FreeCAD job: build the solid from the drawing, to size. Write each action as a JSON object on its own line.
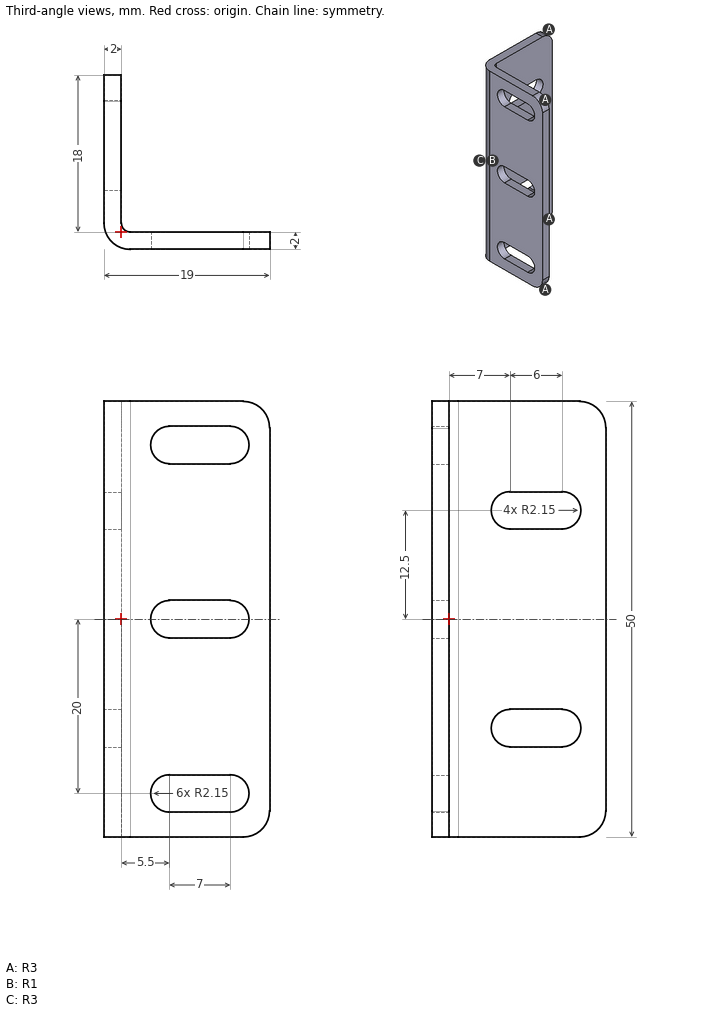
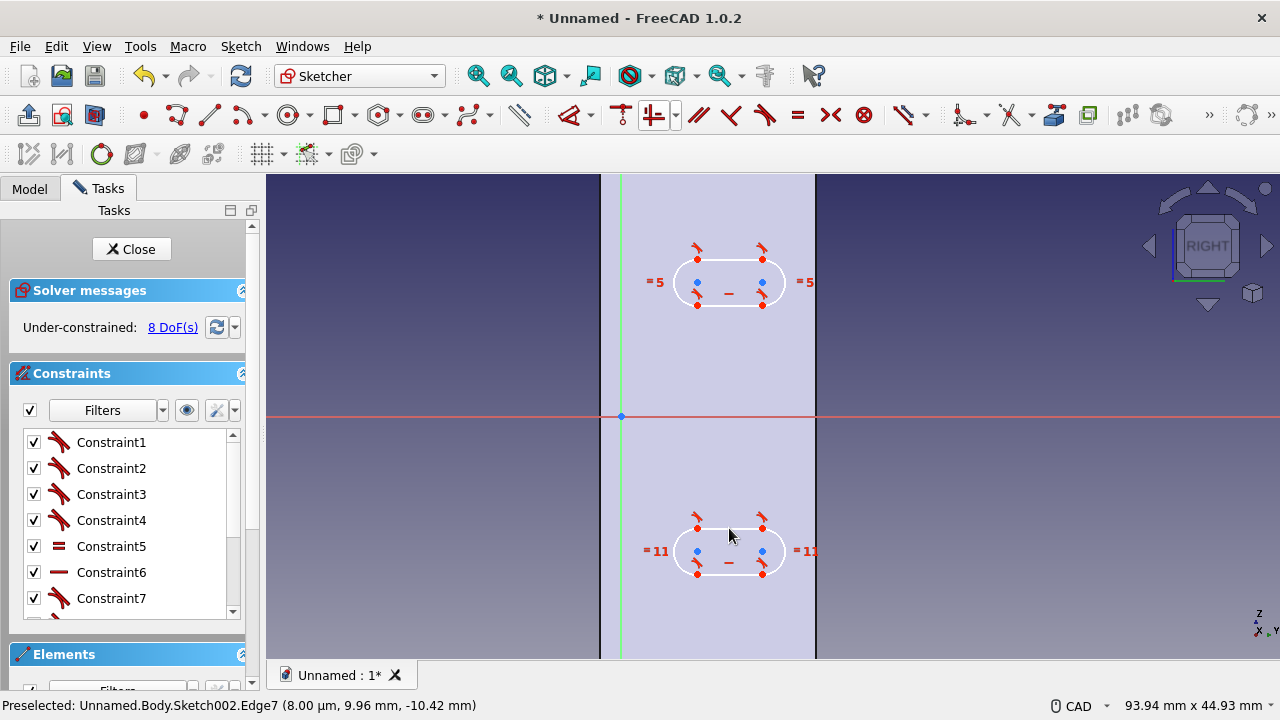
{"action": "left_click", "coordinate": [678, 269]}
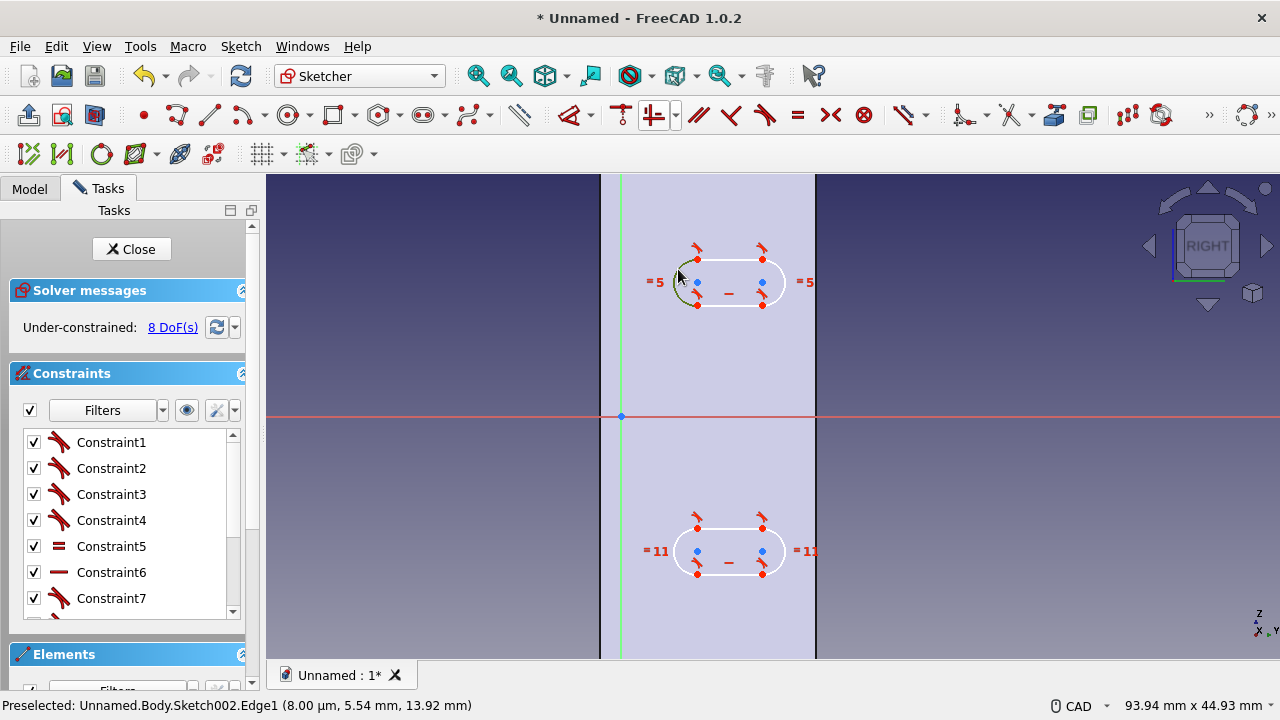
{"action": "left_click", "coordinate": [678, 538]}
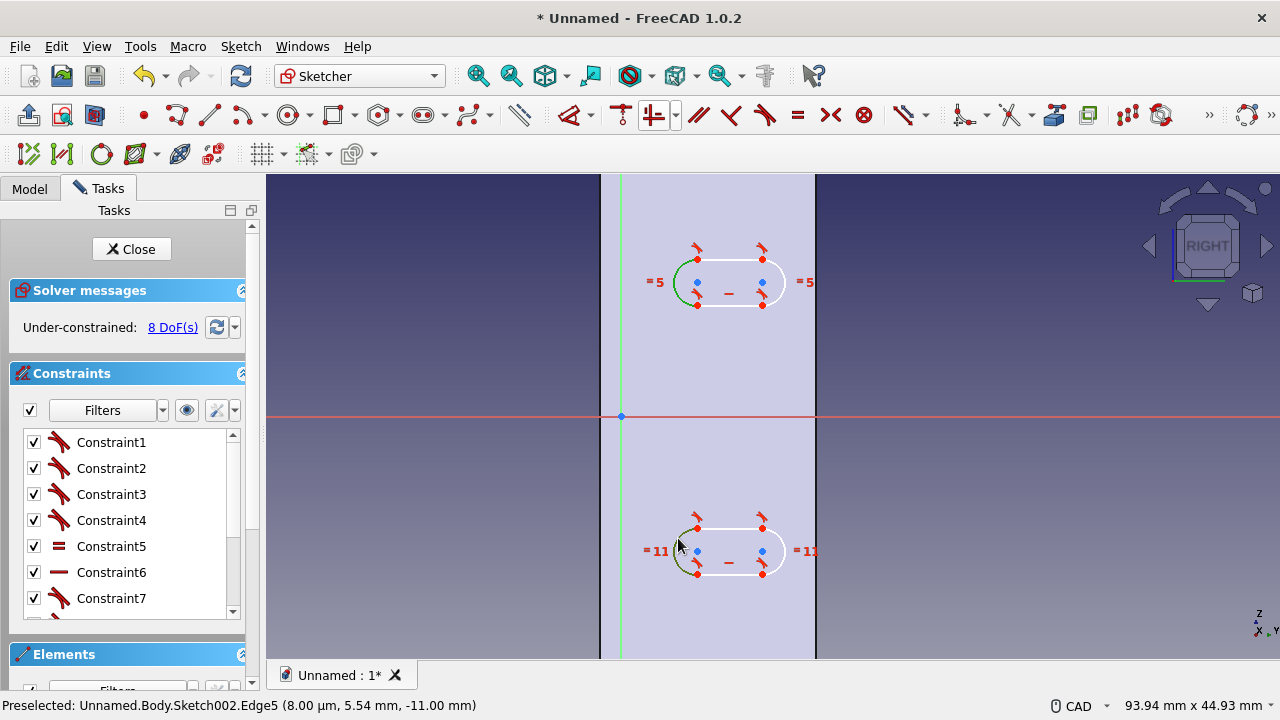
{"action": "left_click", "coordinate": [798, 116]}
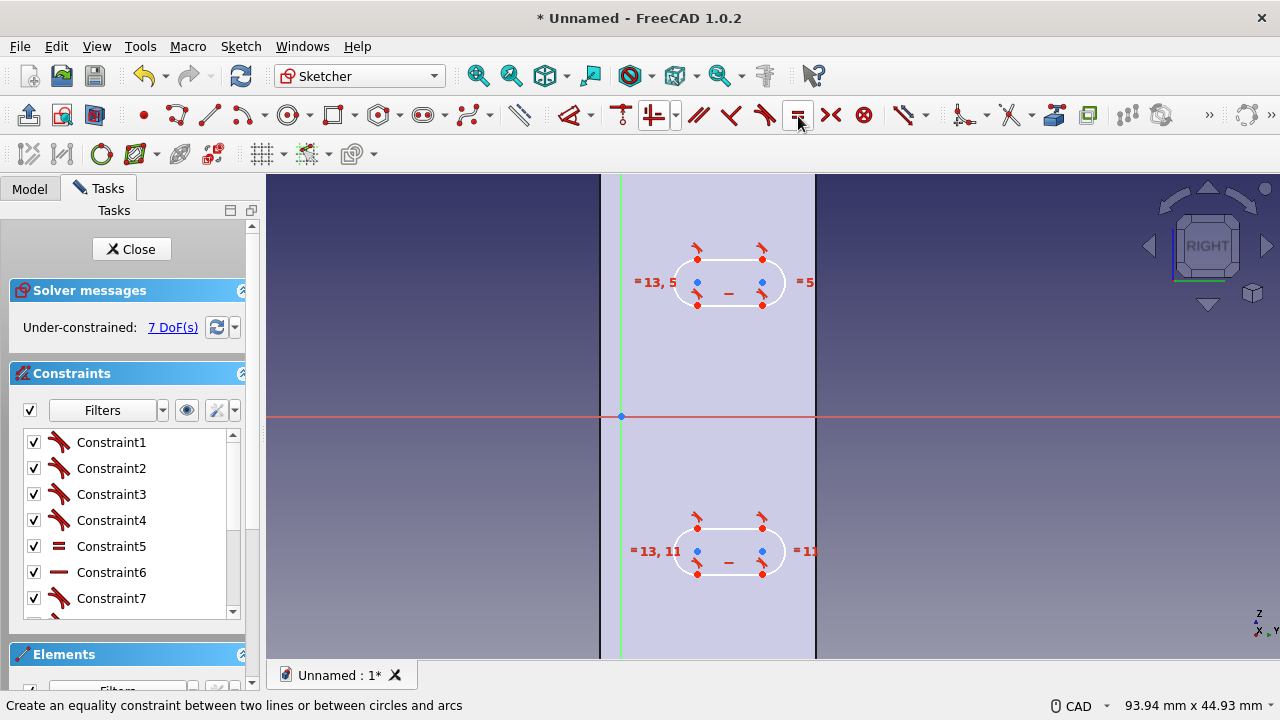
{"action": "left_click", "coordinate": [697, 283]}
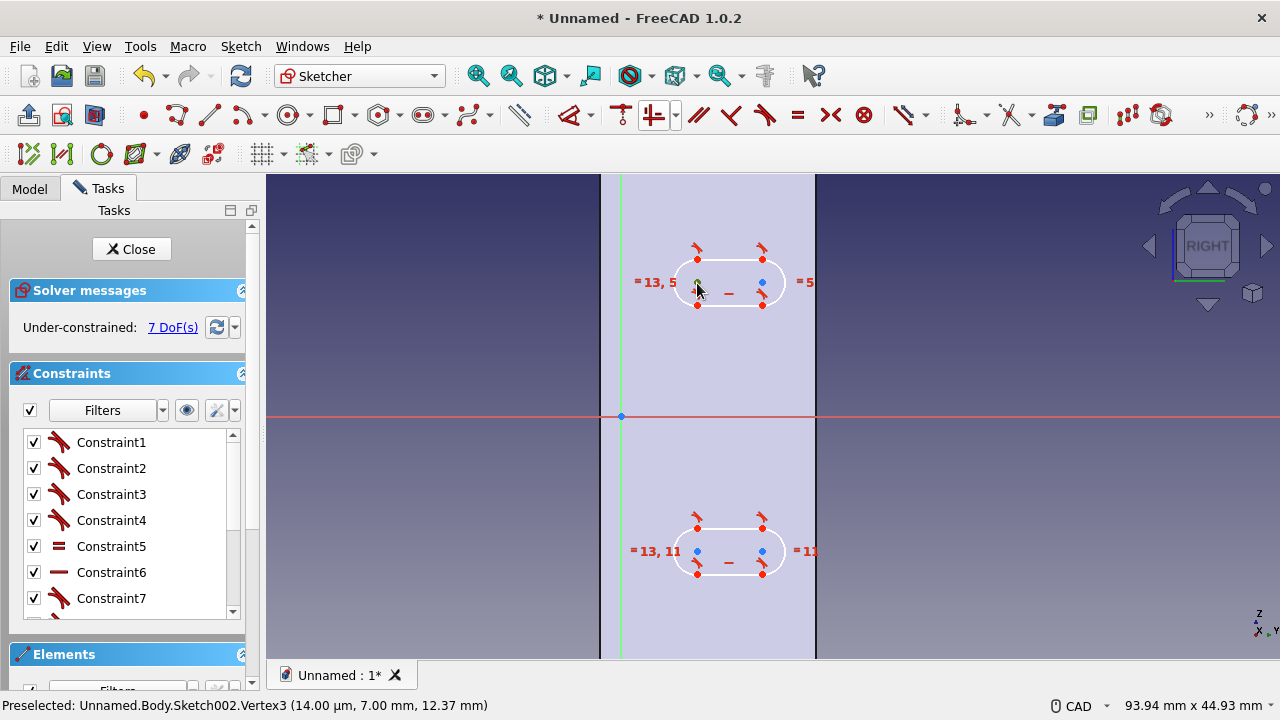
{"action": "left_click", "coordinate": [697, 552]}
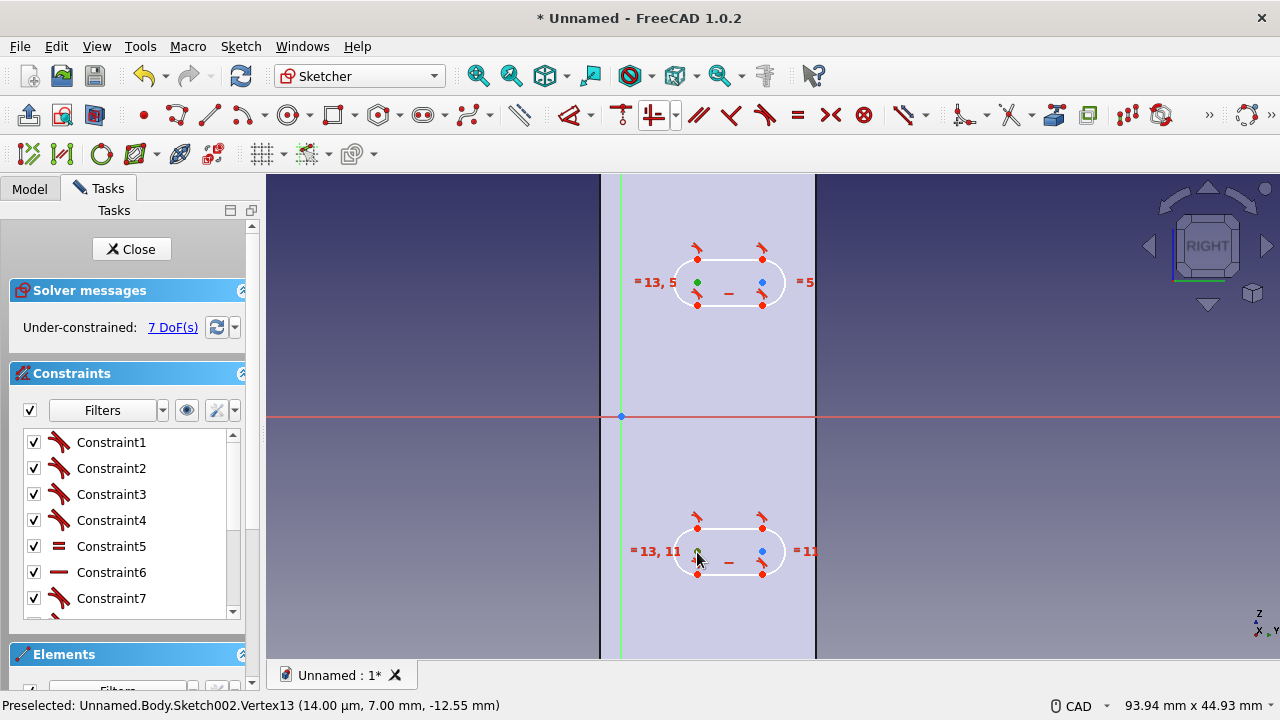
{"action": "left_click", "coordinate": [353, 416]}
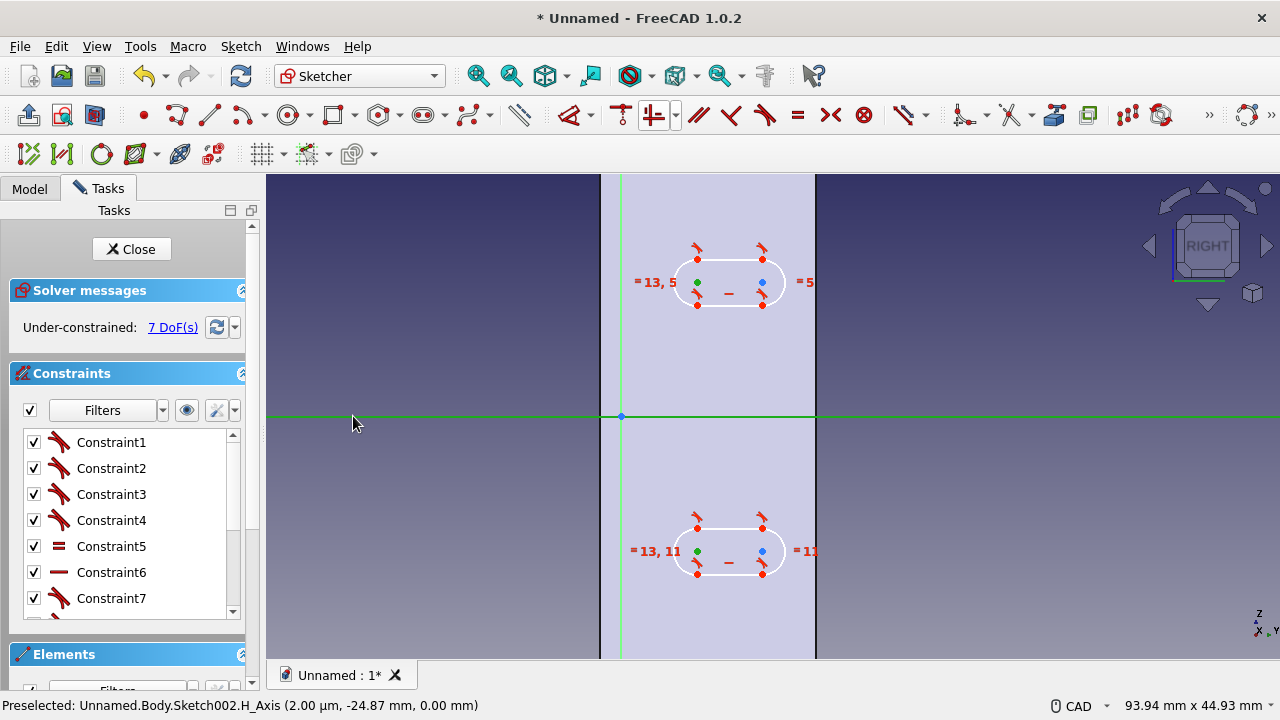
{"action": "left_click", "coordinate": [831, 116]}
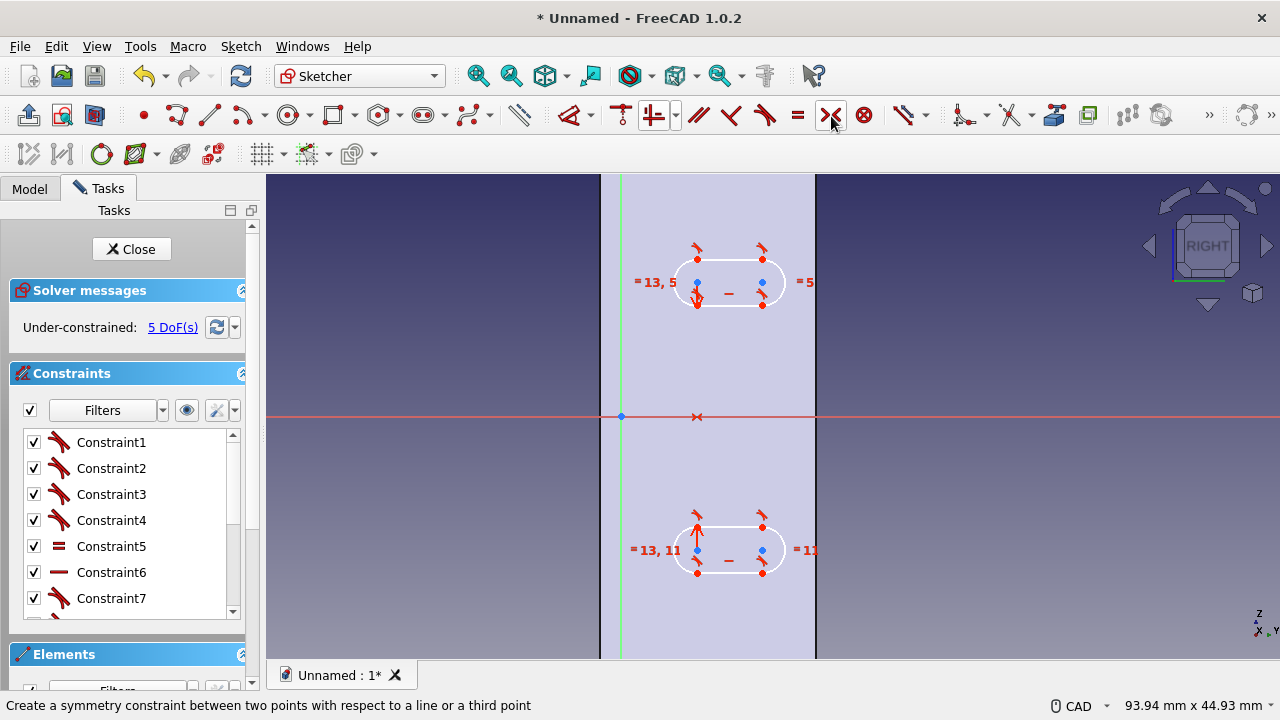
{"action": "left_click", "coordinate": [568, 116]}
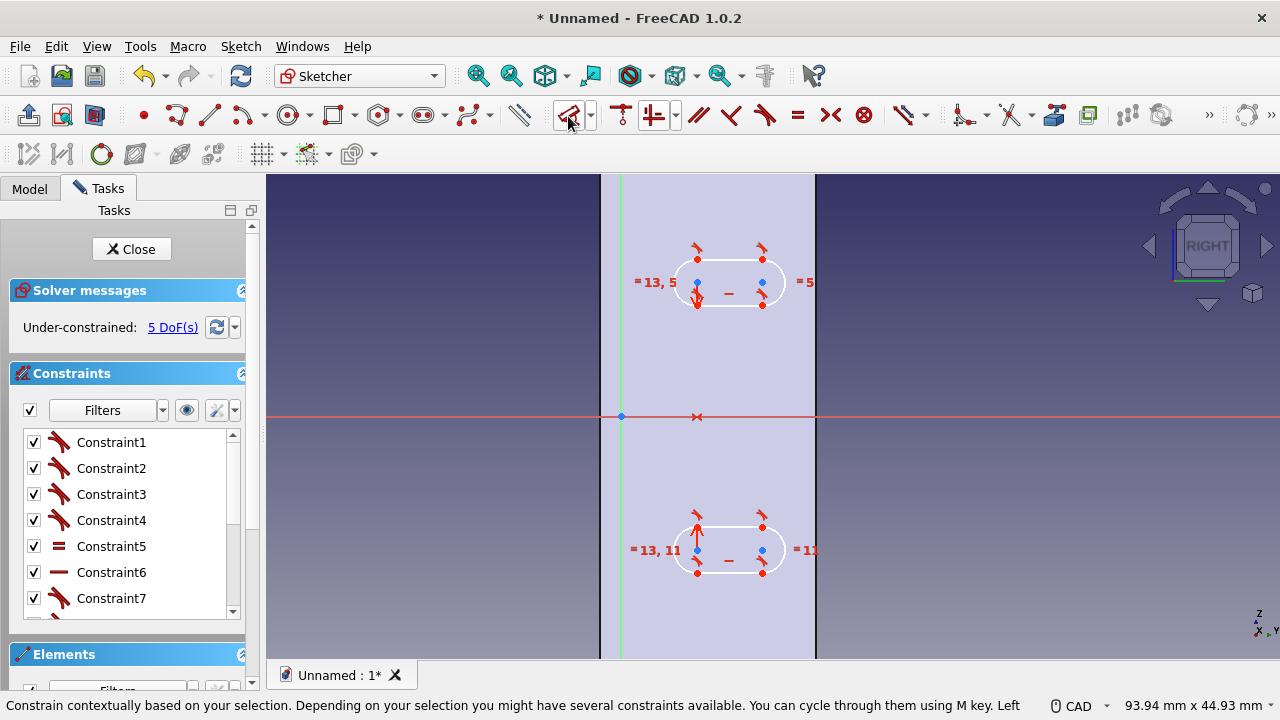
{"action": "scroll", "coordinate": [678, 269], "scroll_direction": "up", "scroll_amount": 3}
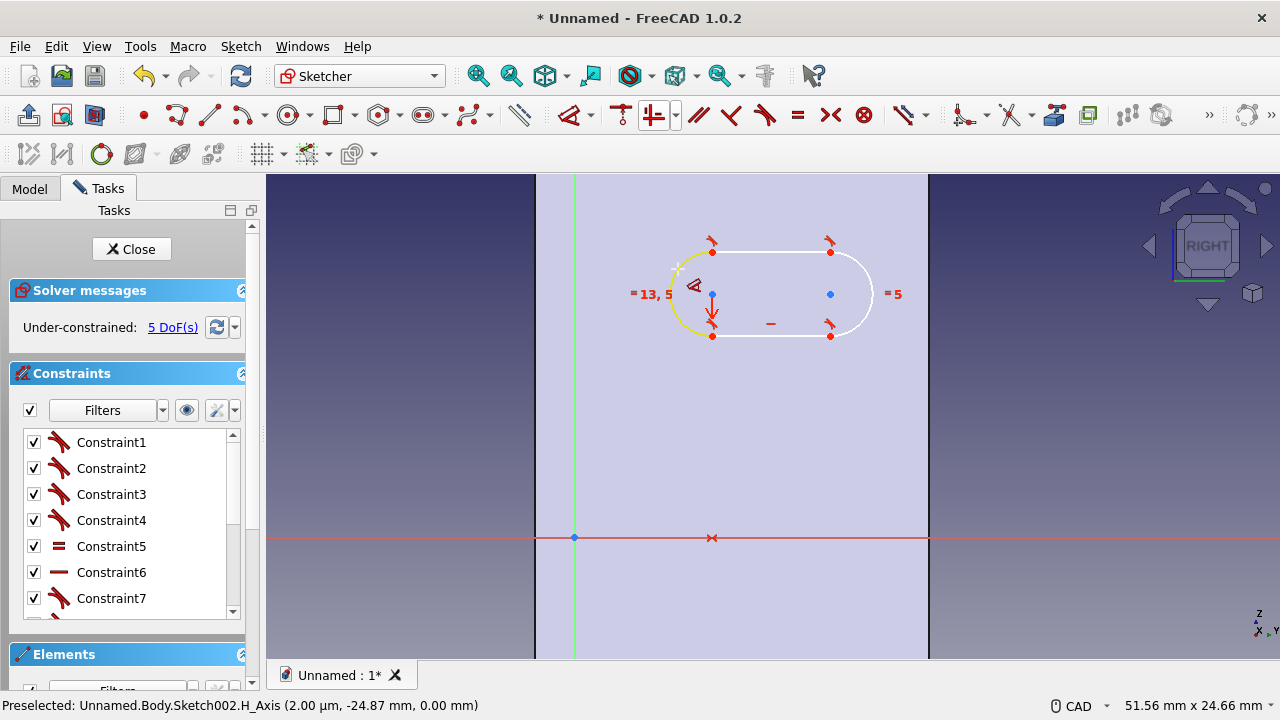
{"action": "left_click", "coordinate": [678, 270]}
{"action": "left_click", "coordinate": [652, 252]}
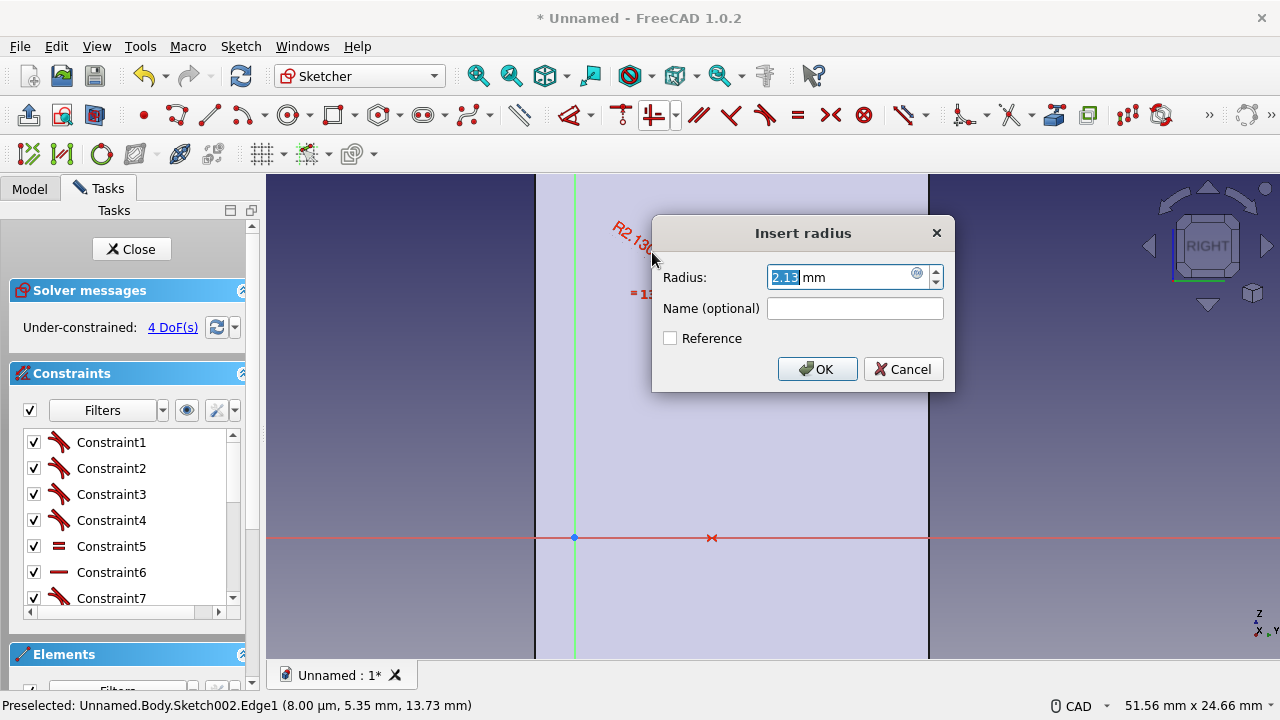
{"action": "type", "text": "2.15"}
{"action": "key", "text": "Return"}